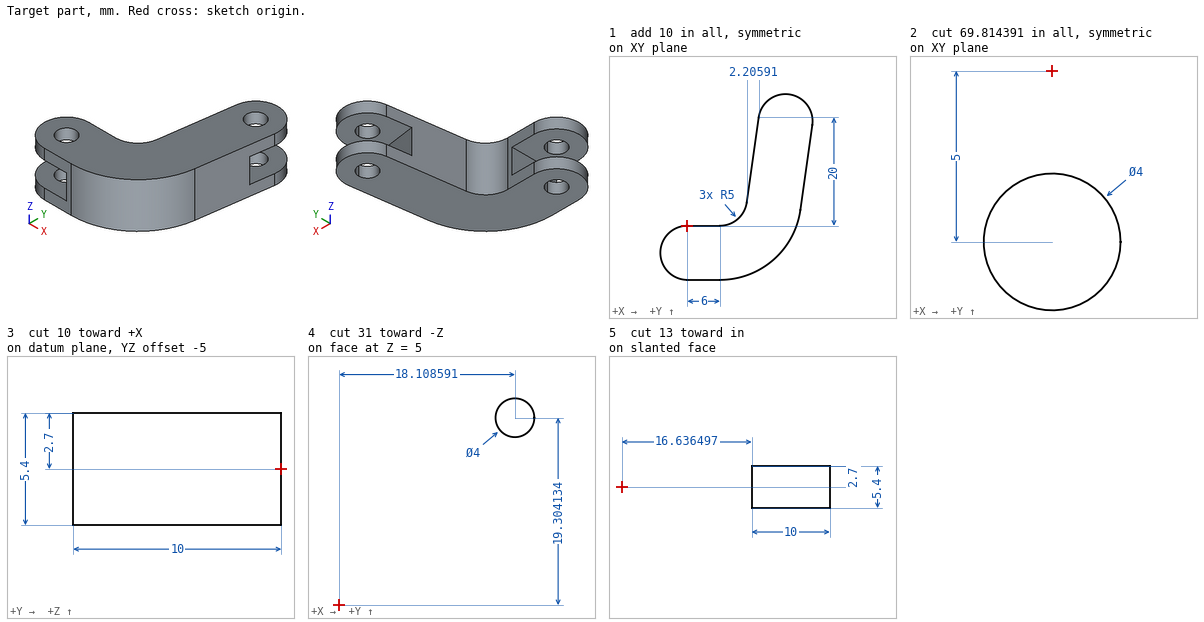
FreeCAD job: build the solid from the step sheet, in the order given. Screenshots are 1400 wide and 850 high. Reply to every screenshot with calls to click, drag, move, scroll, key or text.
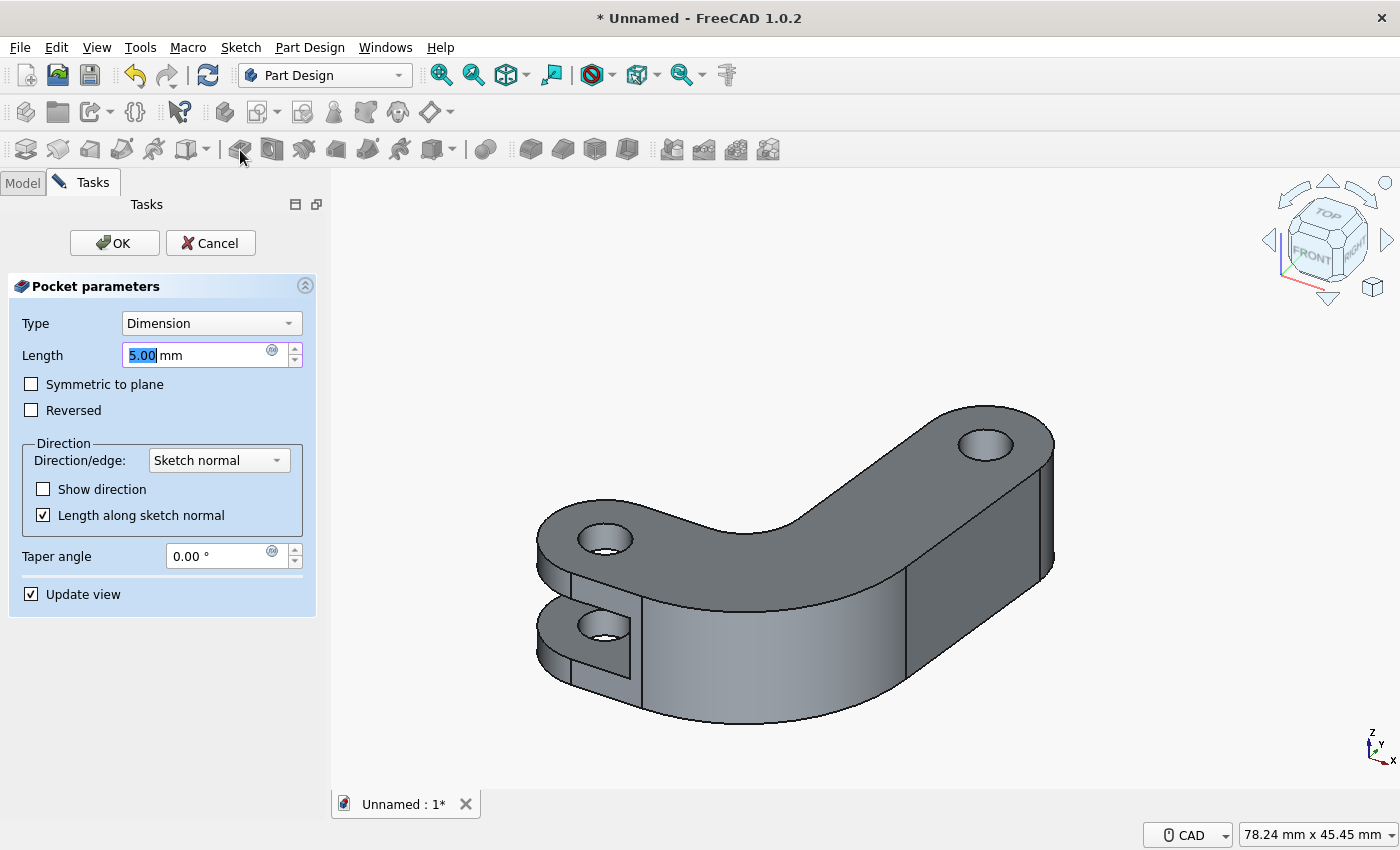
text(31)
key(Tab)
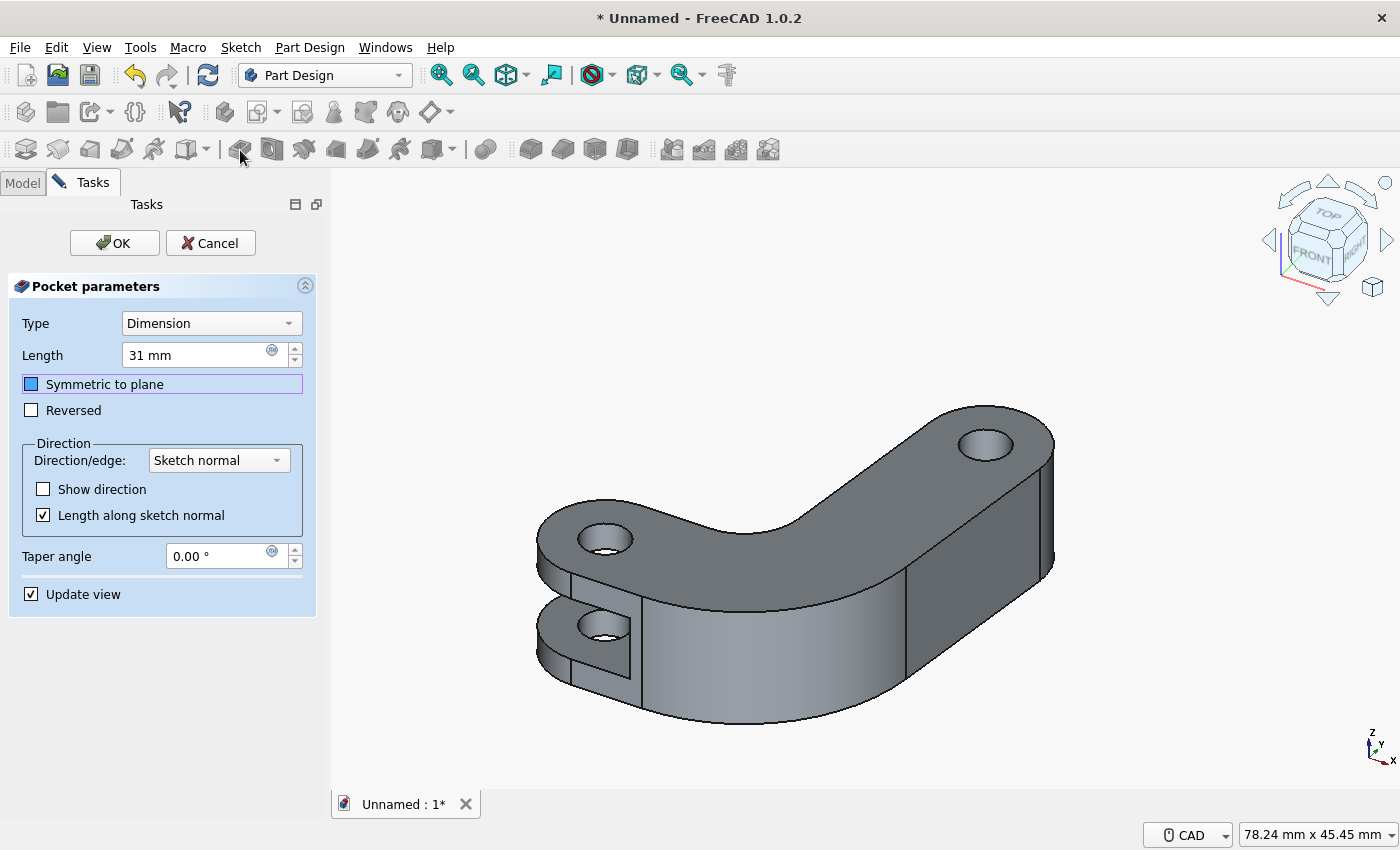
click(115, 243)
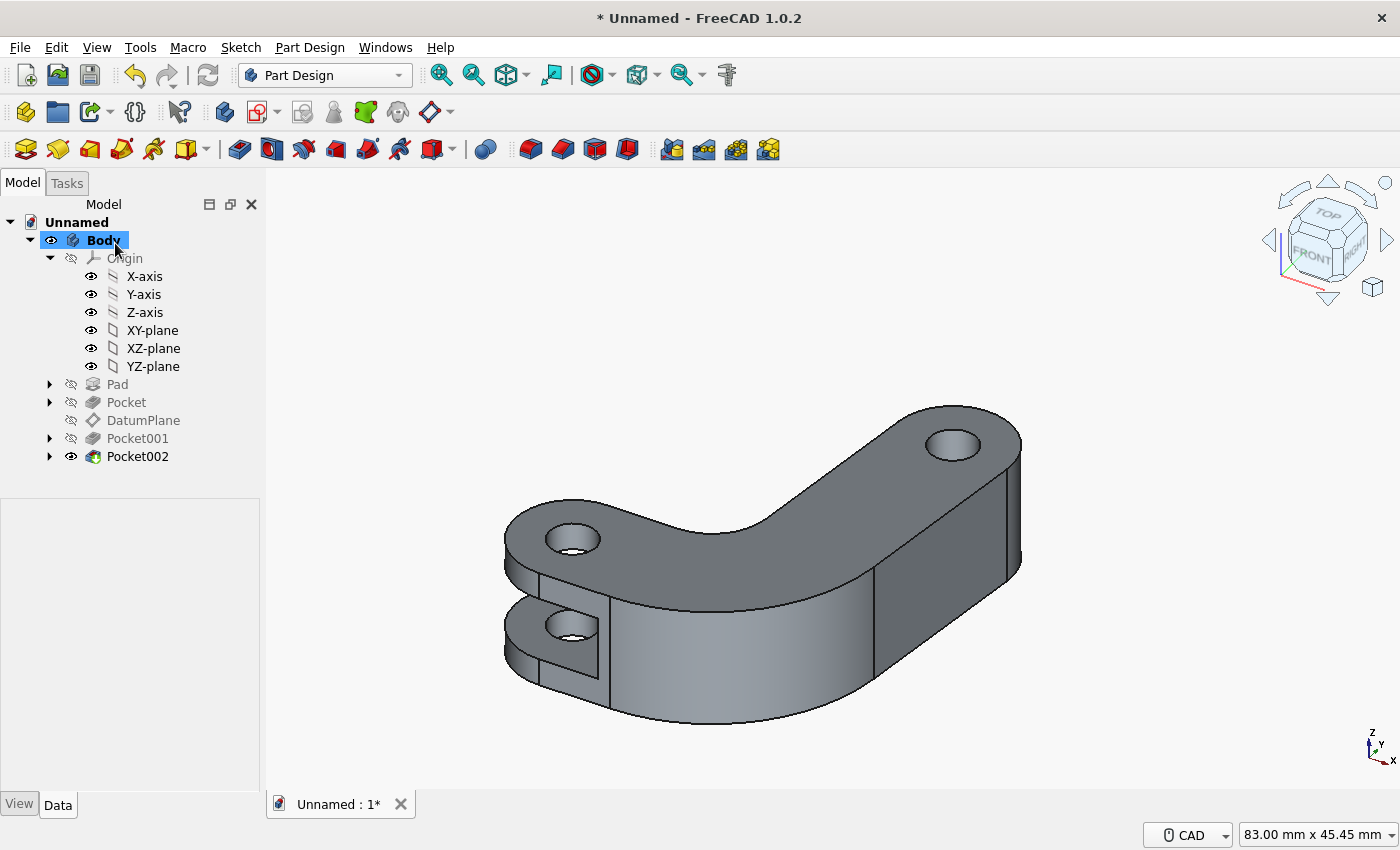
click(959, 559)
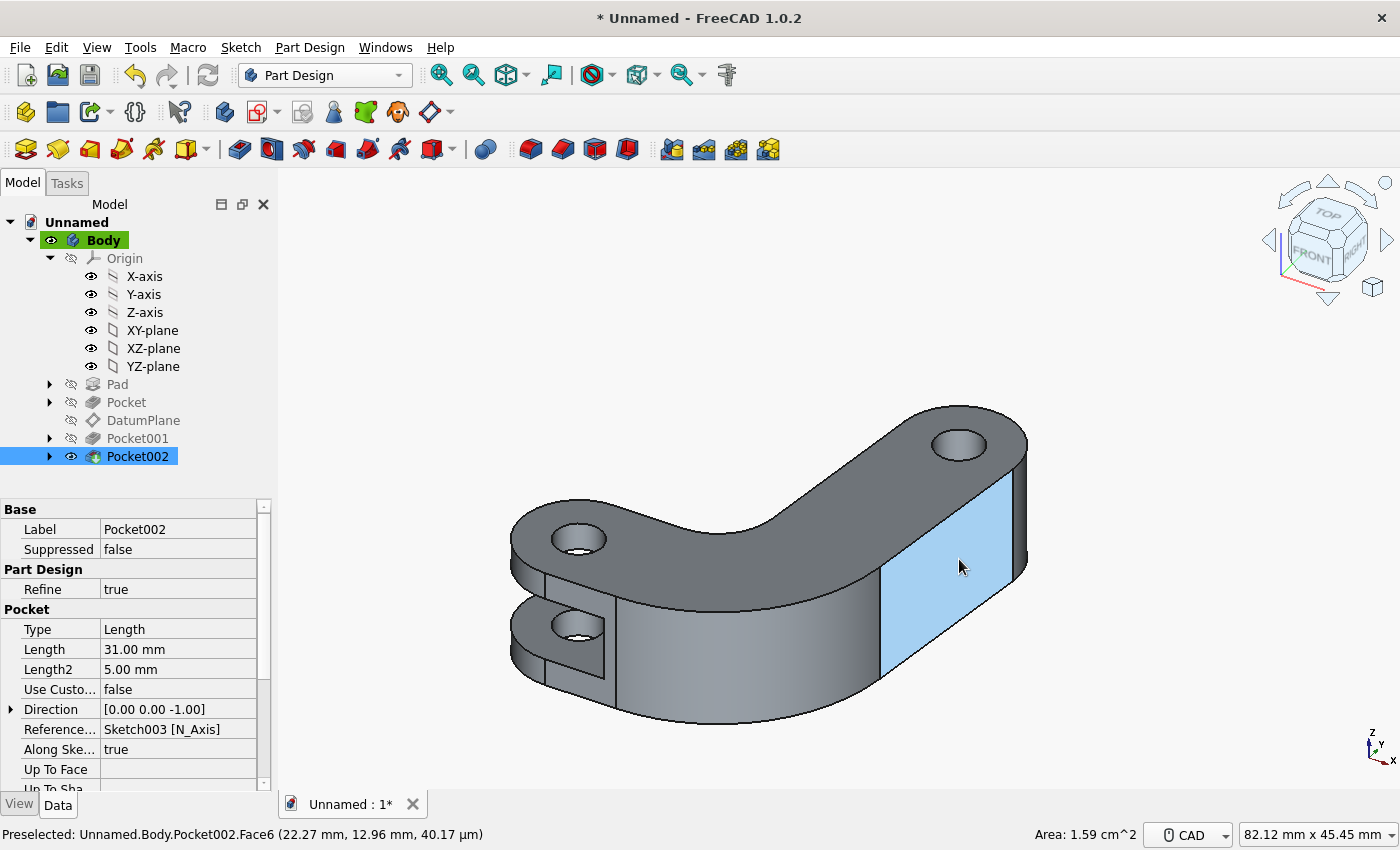
click(258, 112)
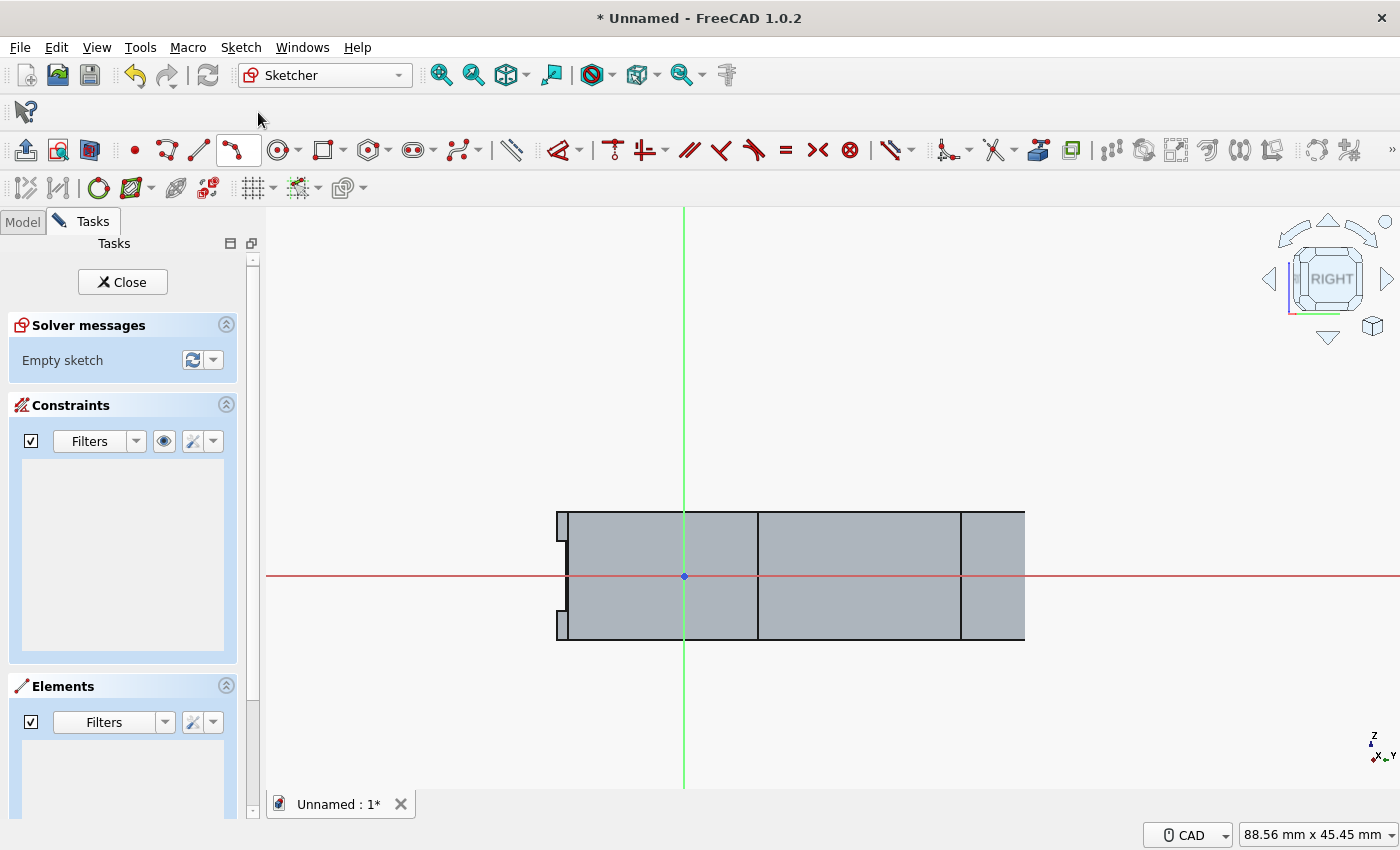
scroll(1011, 596, up, 8)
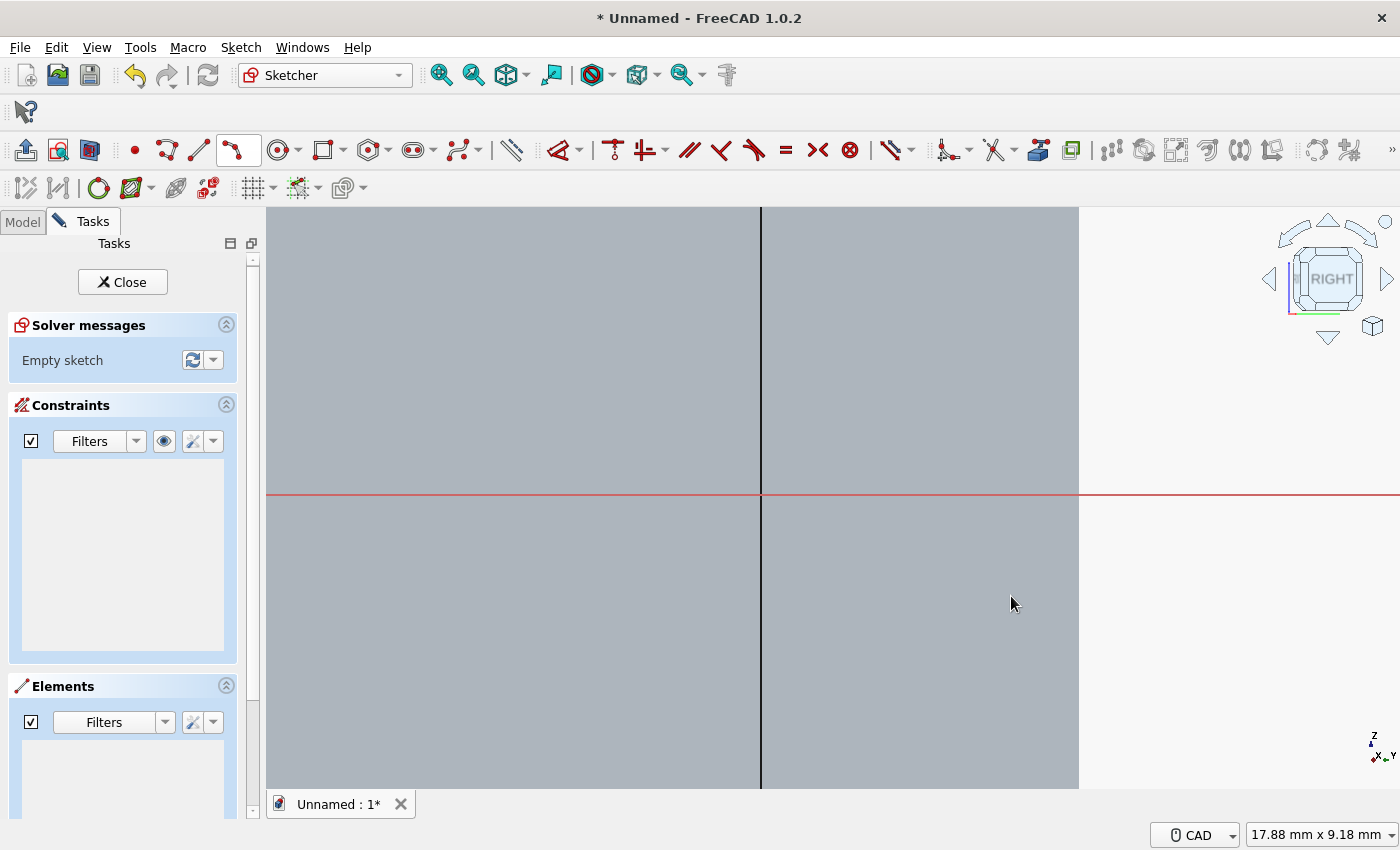
click(324, 150)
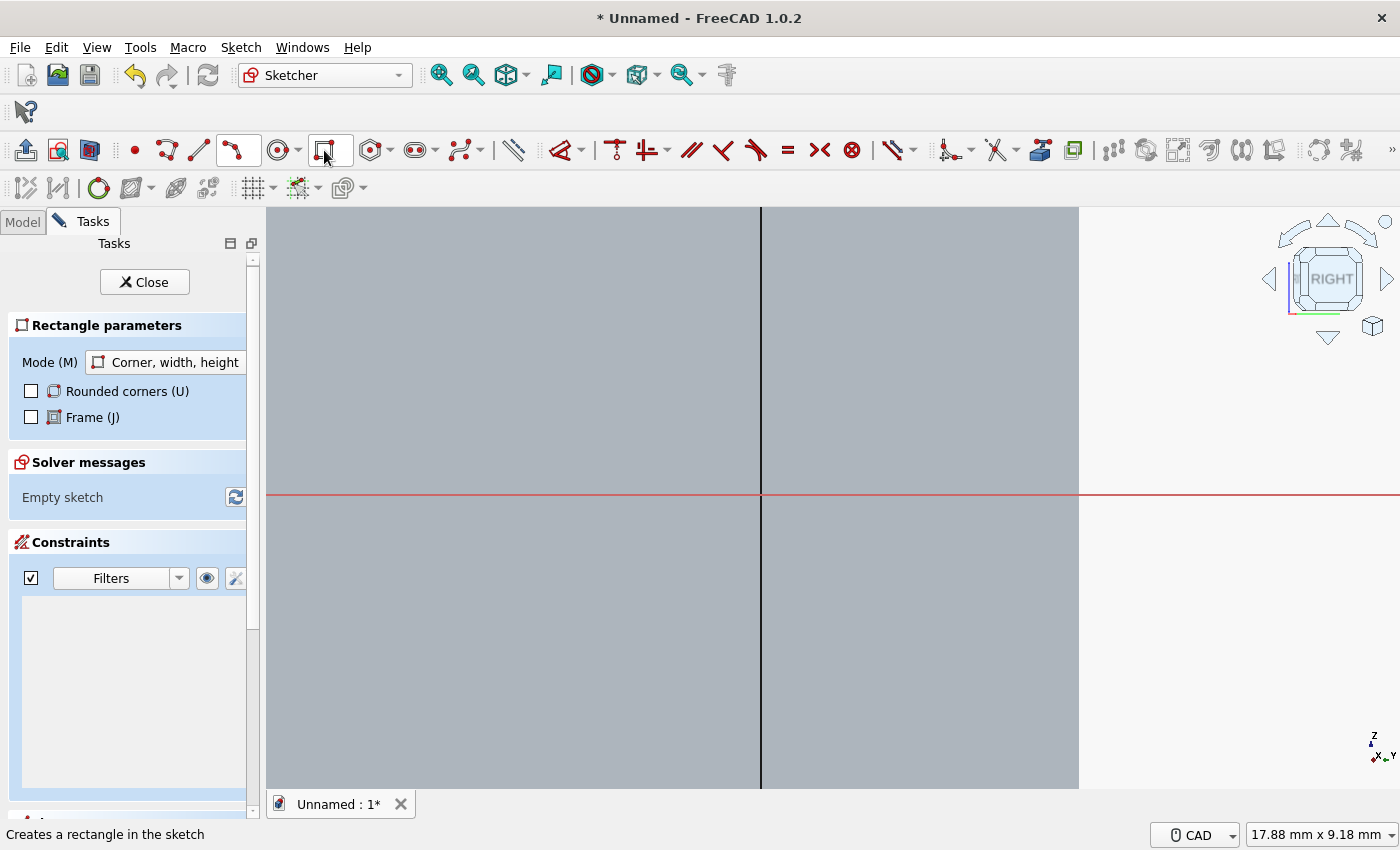
click(444, 323)
click(1079, 666)
key(Escape)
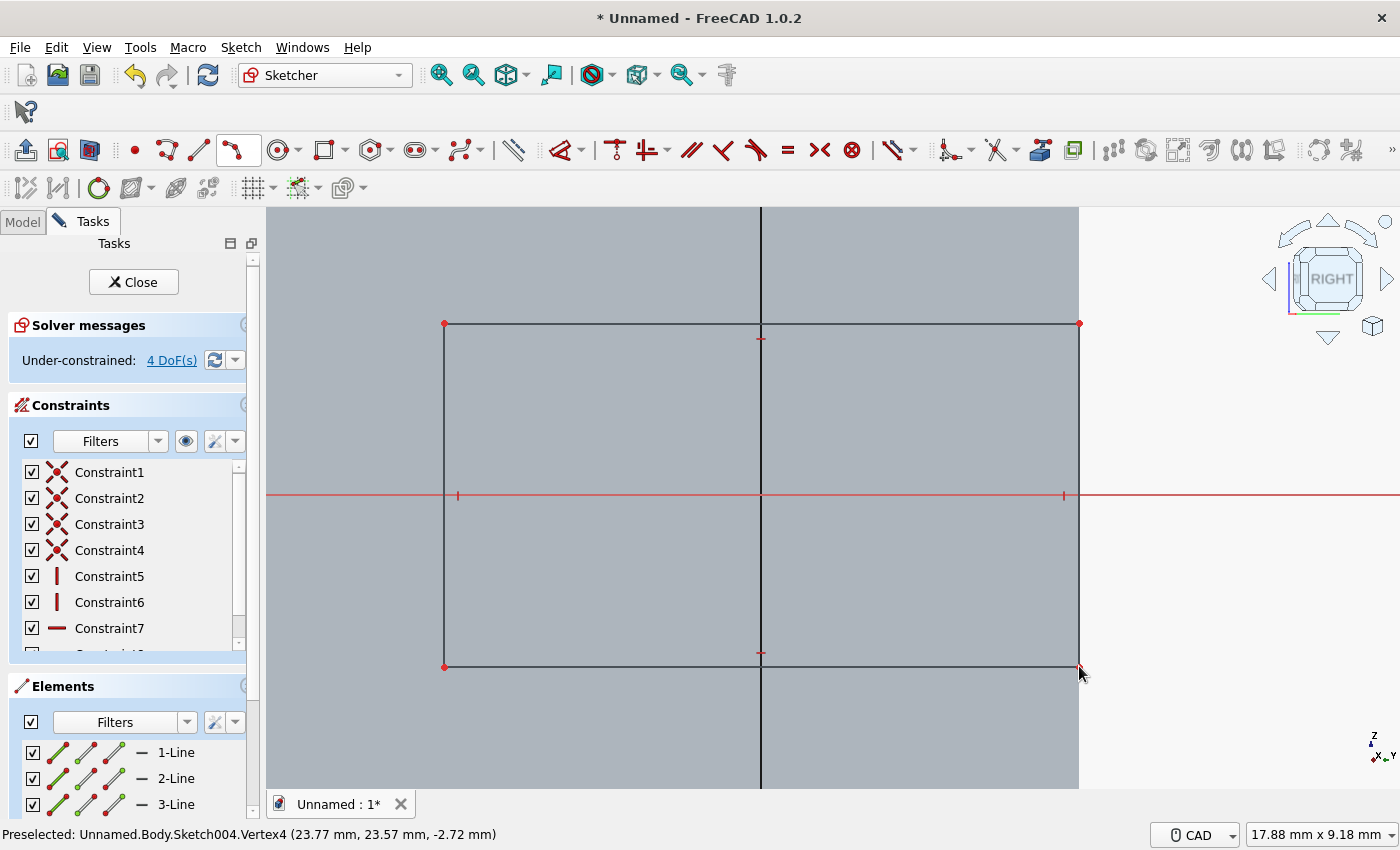
click(560, 150)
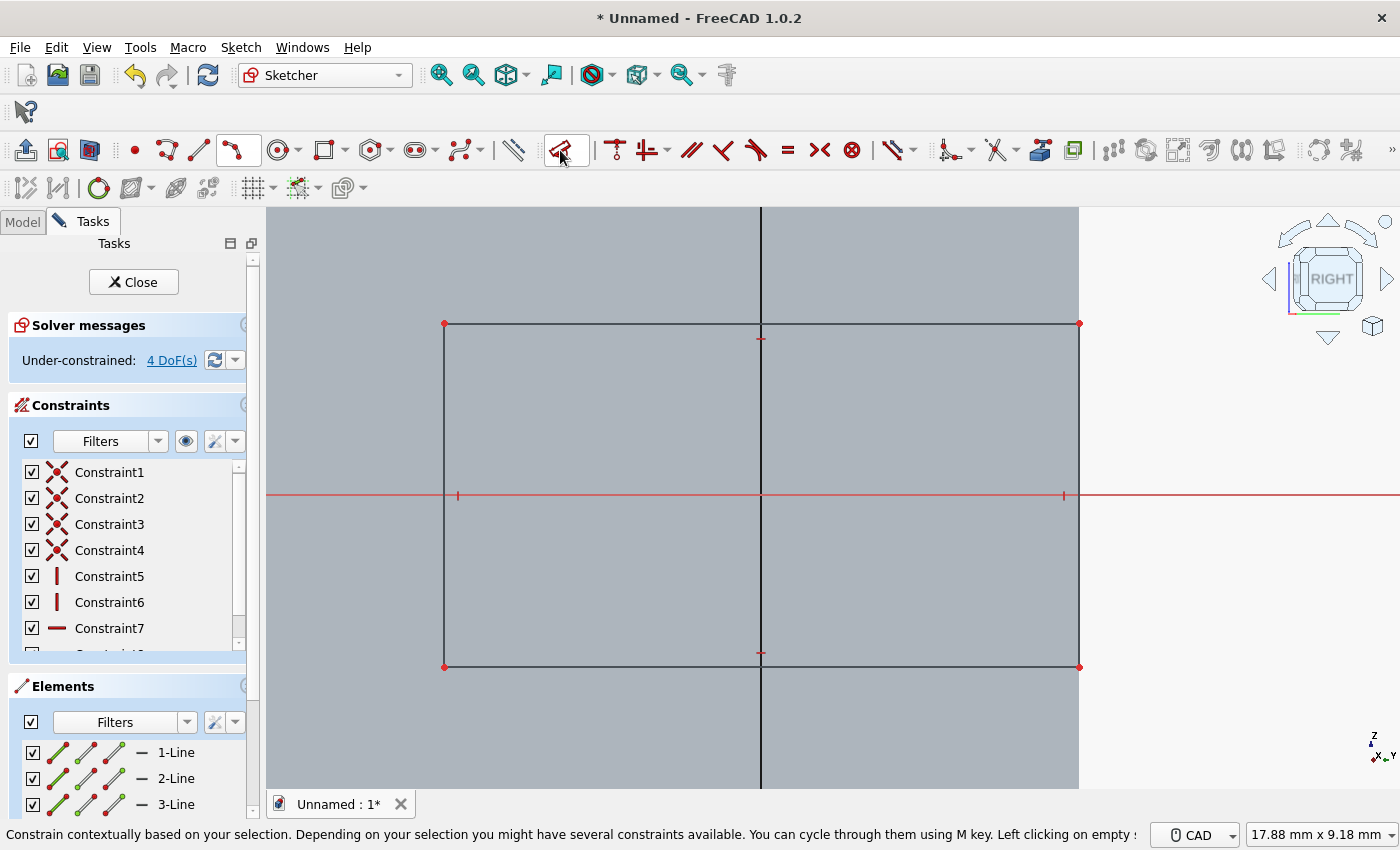
click(635, 667)
click(762, 701)